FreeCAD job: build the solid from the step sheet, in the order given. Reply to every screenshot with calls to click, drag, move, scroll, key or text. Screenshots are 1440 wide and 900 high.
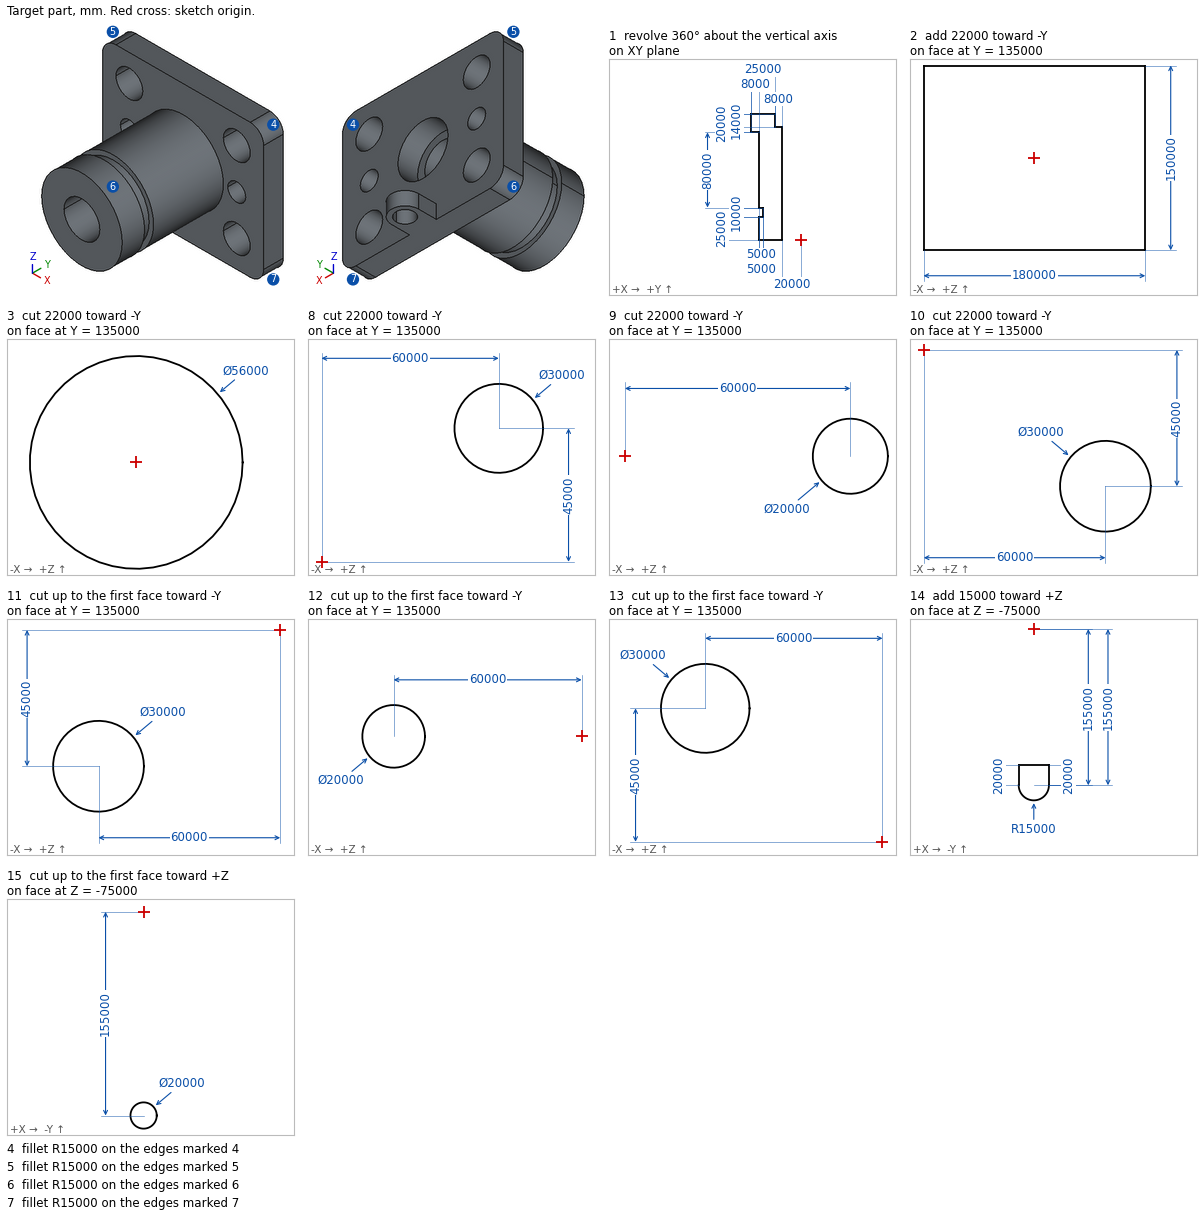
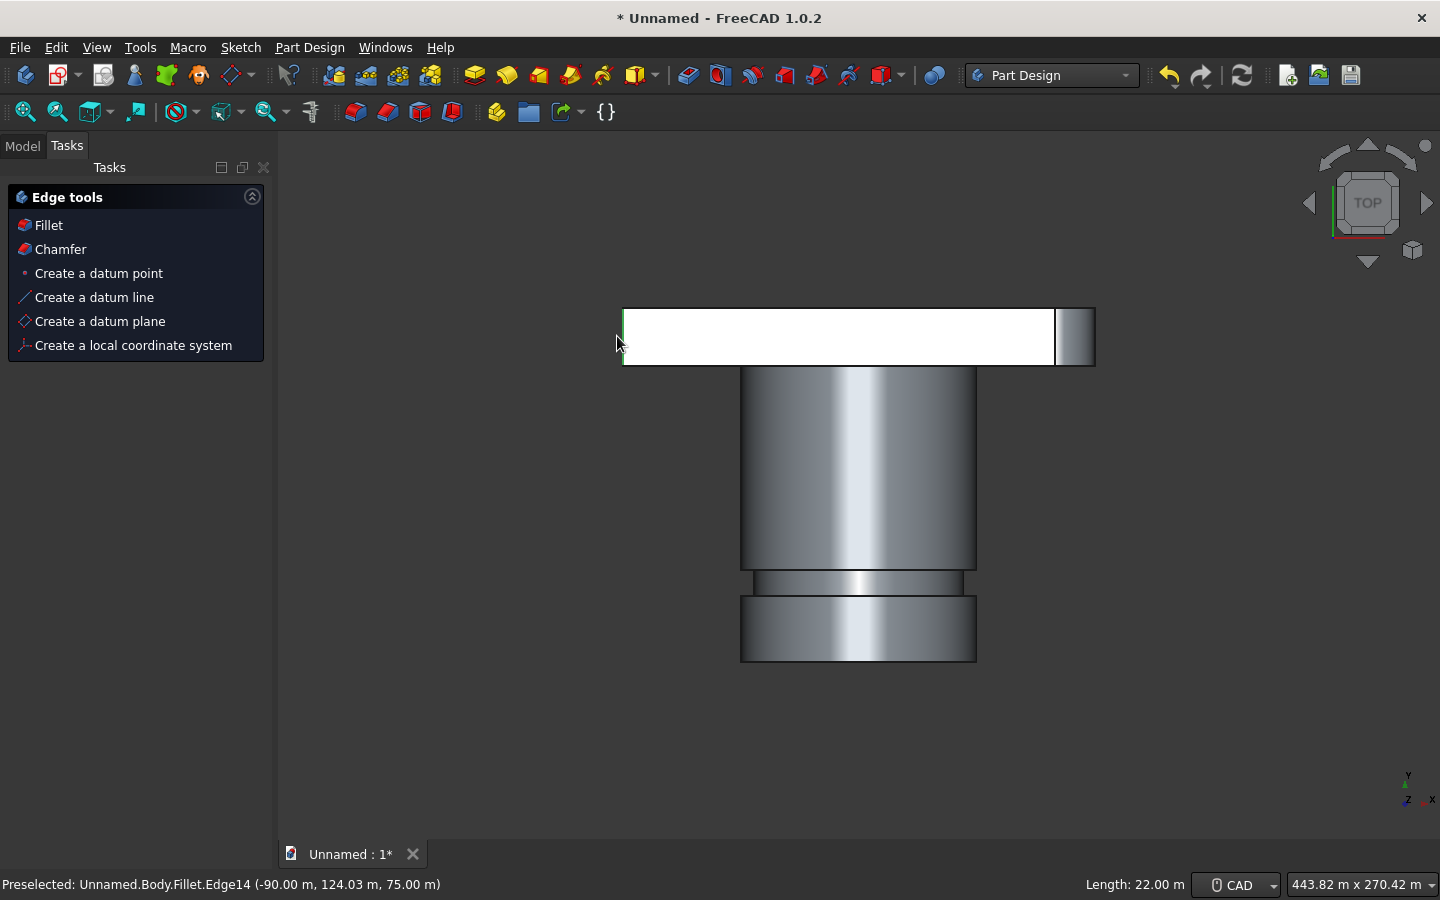
click(356, 112)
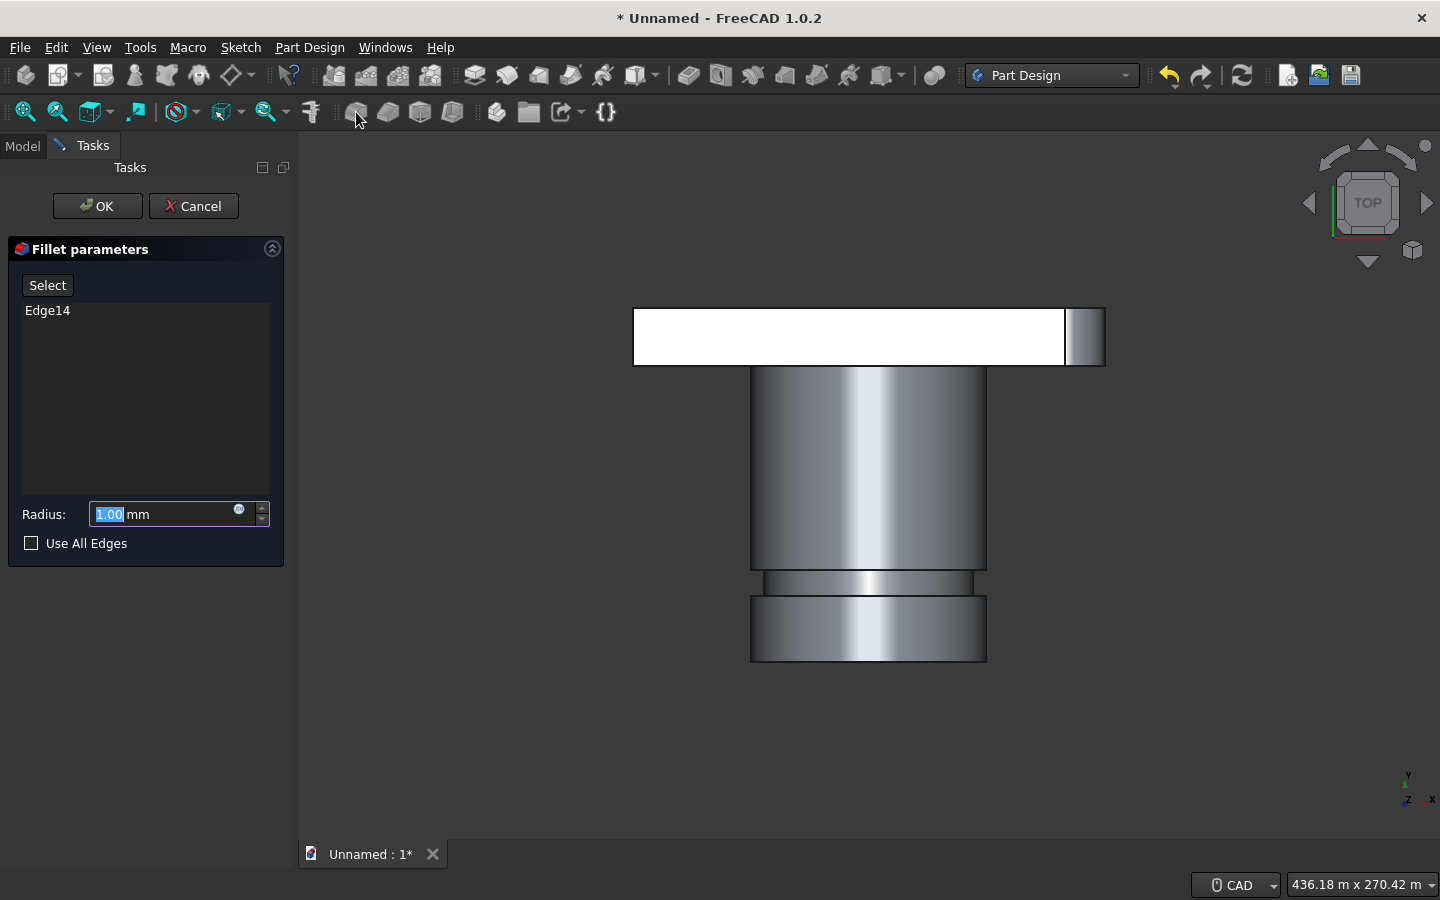
text(15000)
key(Tab)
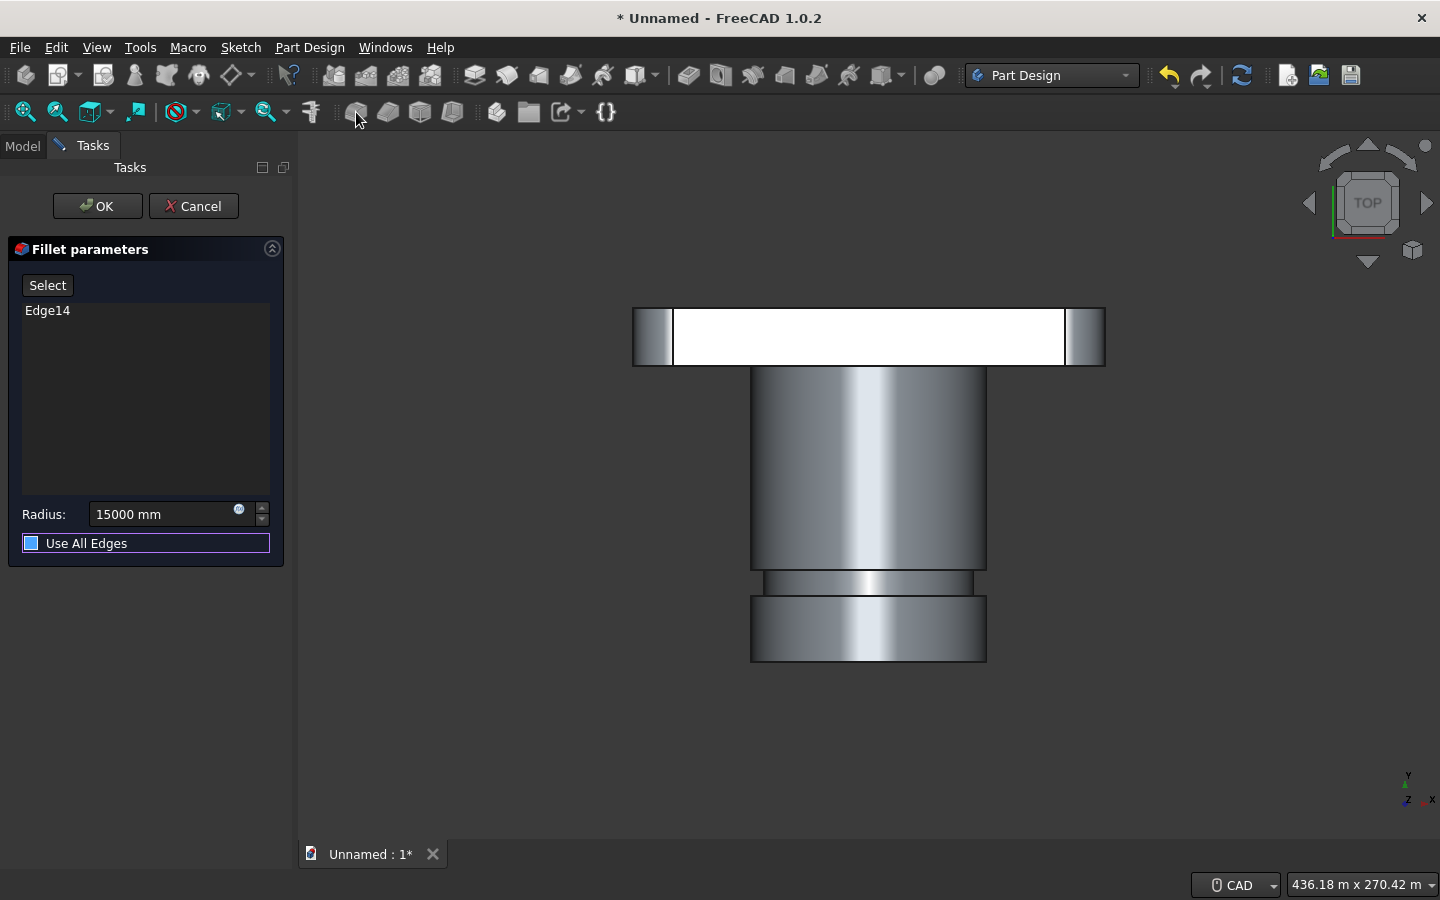
click(98, 206)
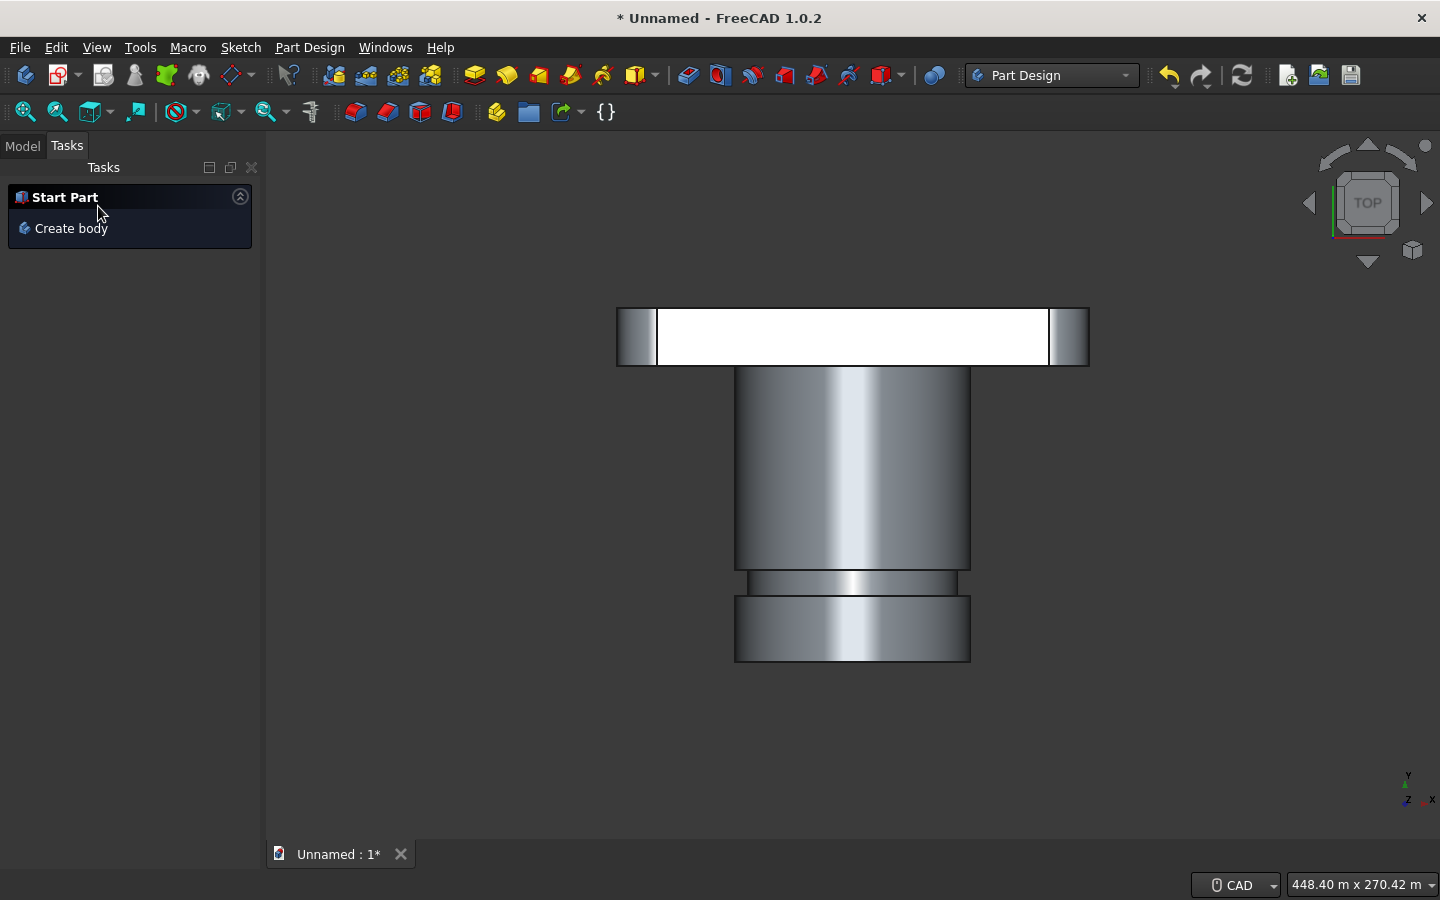
key(0)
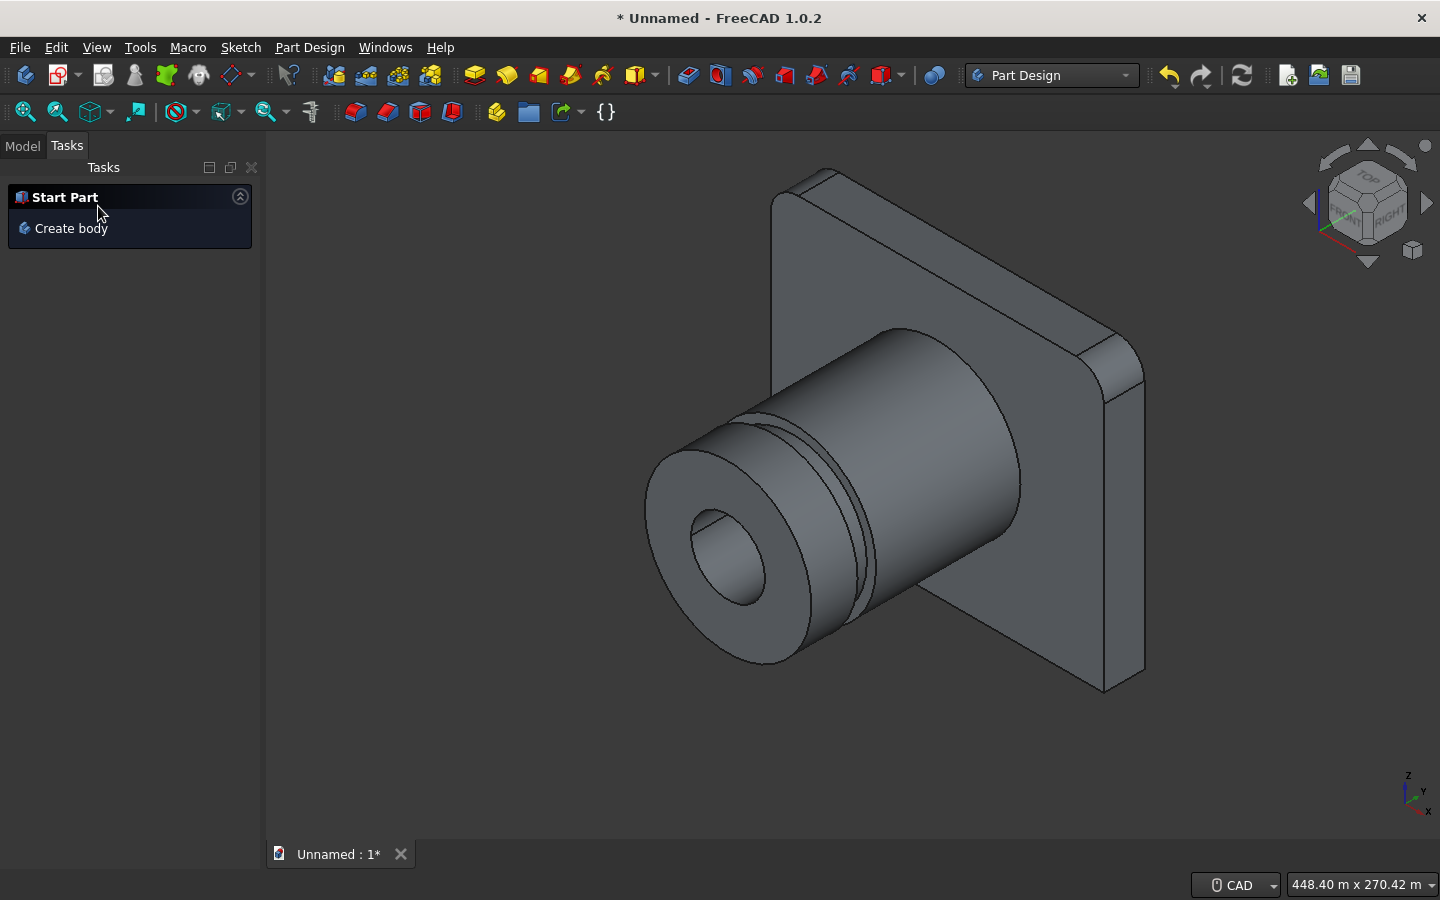
key(2)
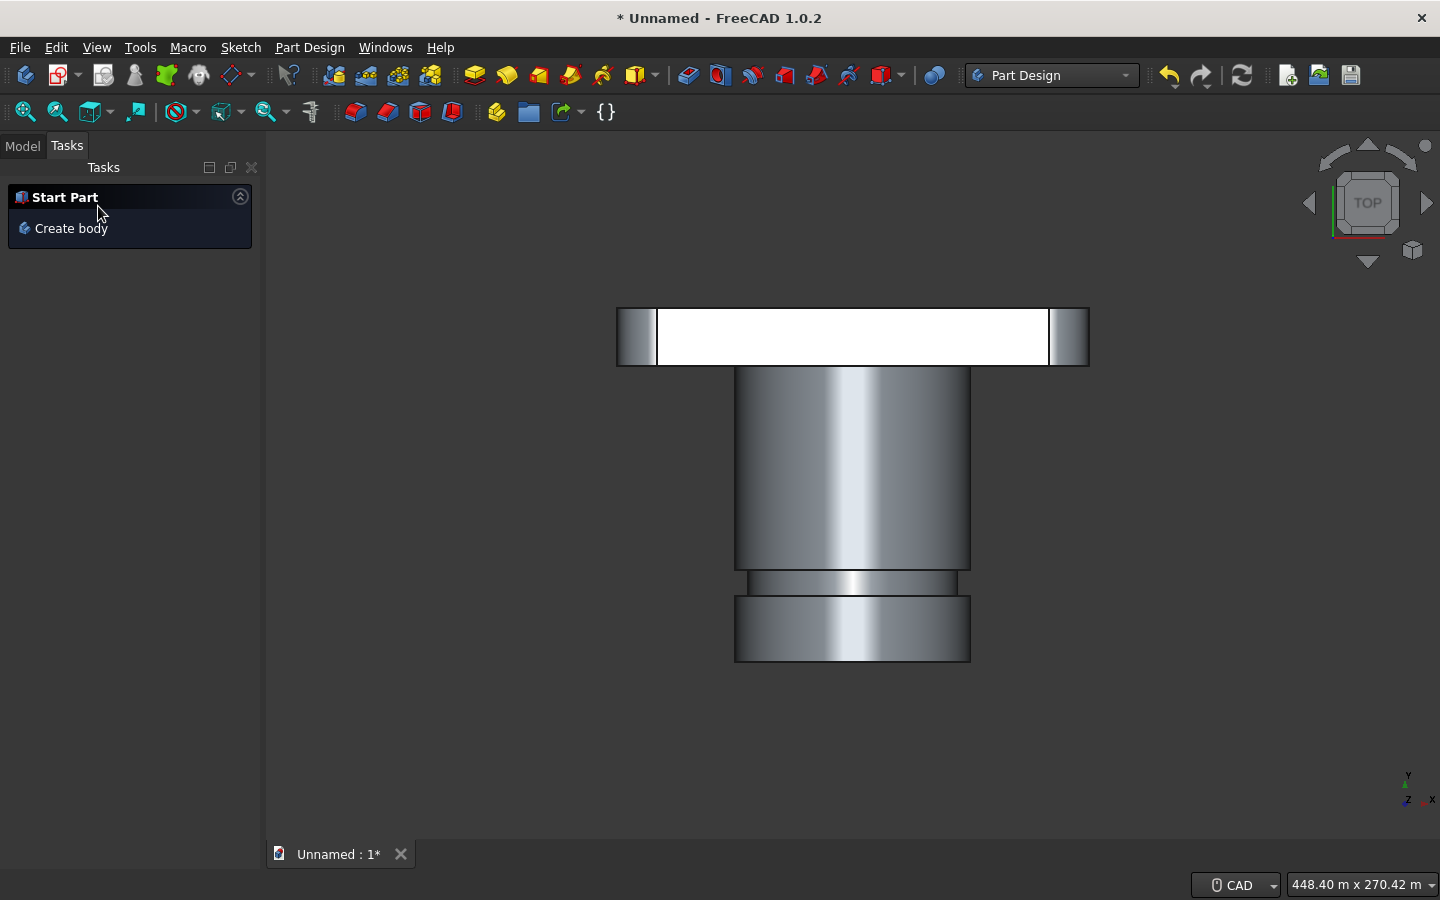
key(1)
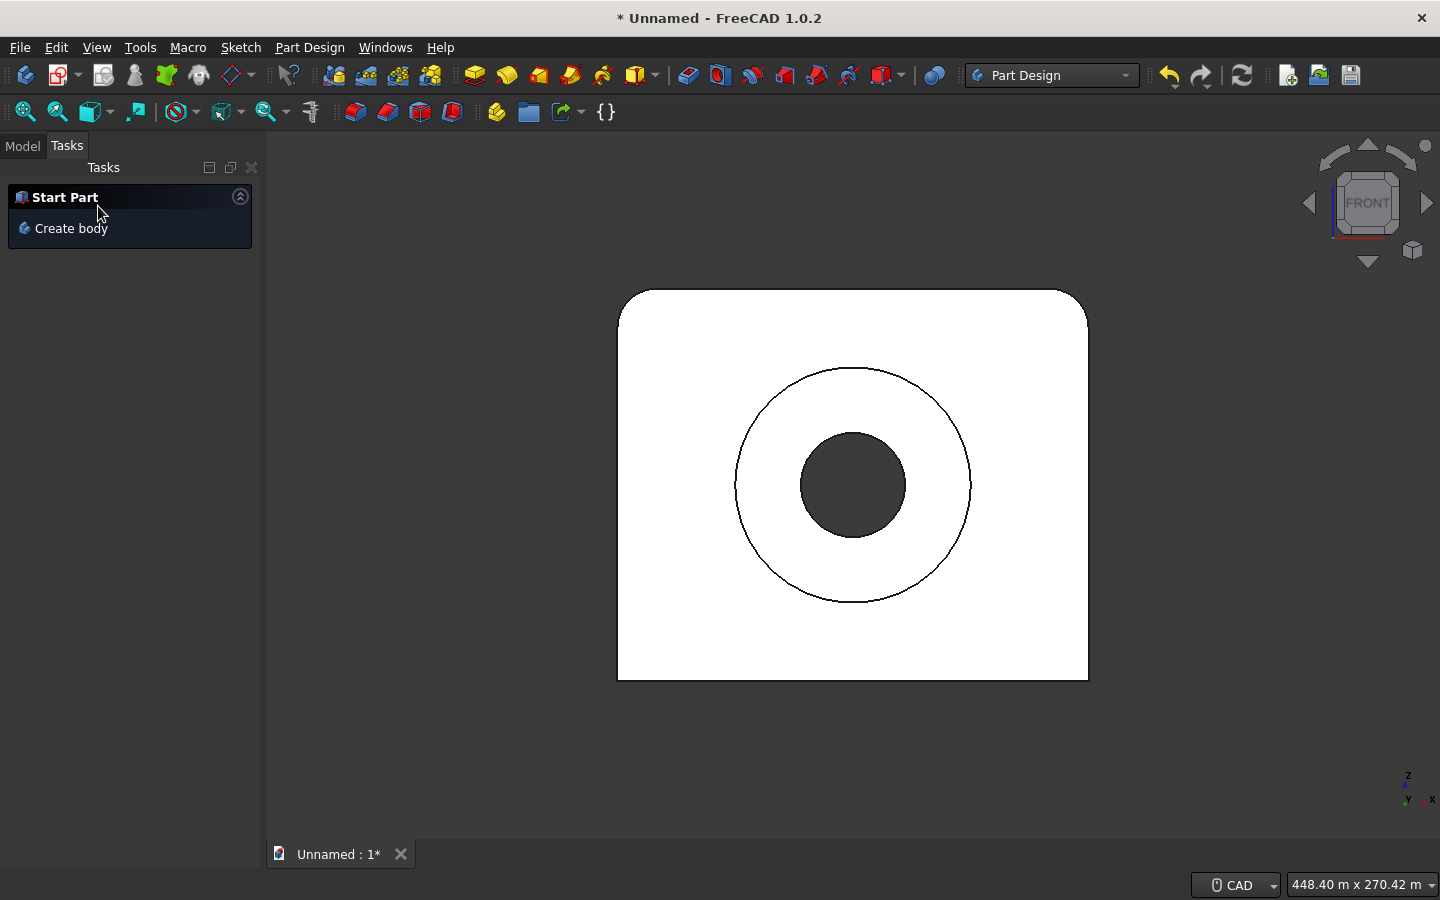
key(3)